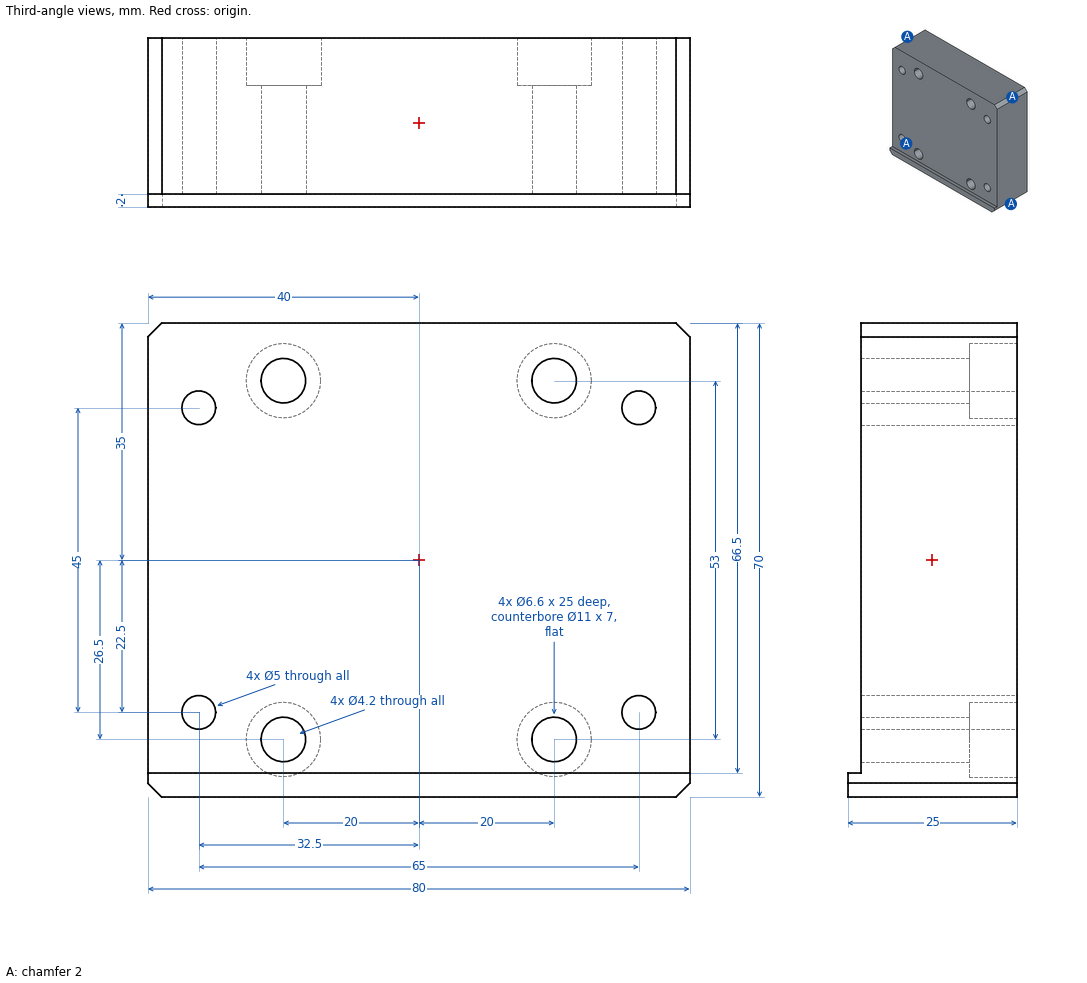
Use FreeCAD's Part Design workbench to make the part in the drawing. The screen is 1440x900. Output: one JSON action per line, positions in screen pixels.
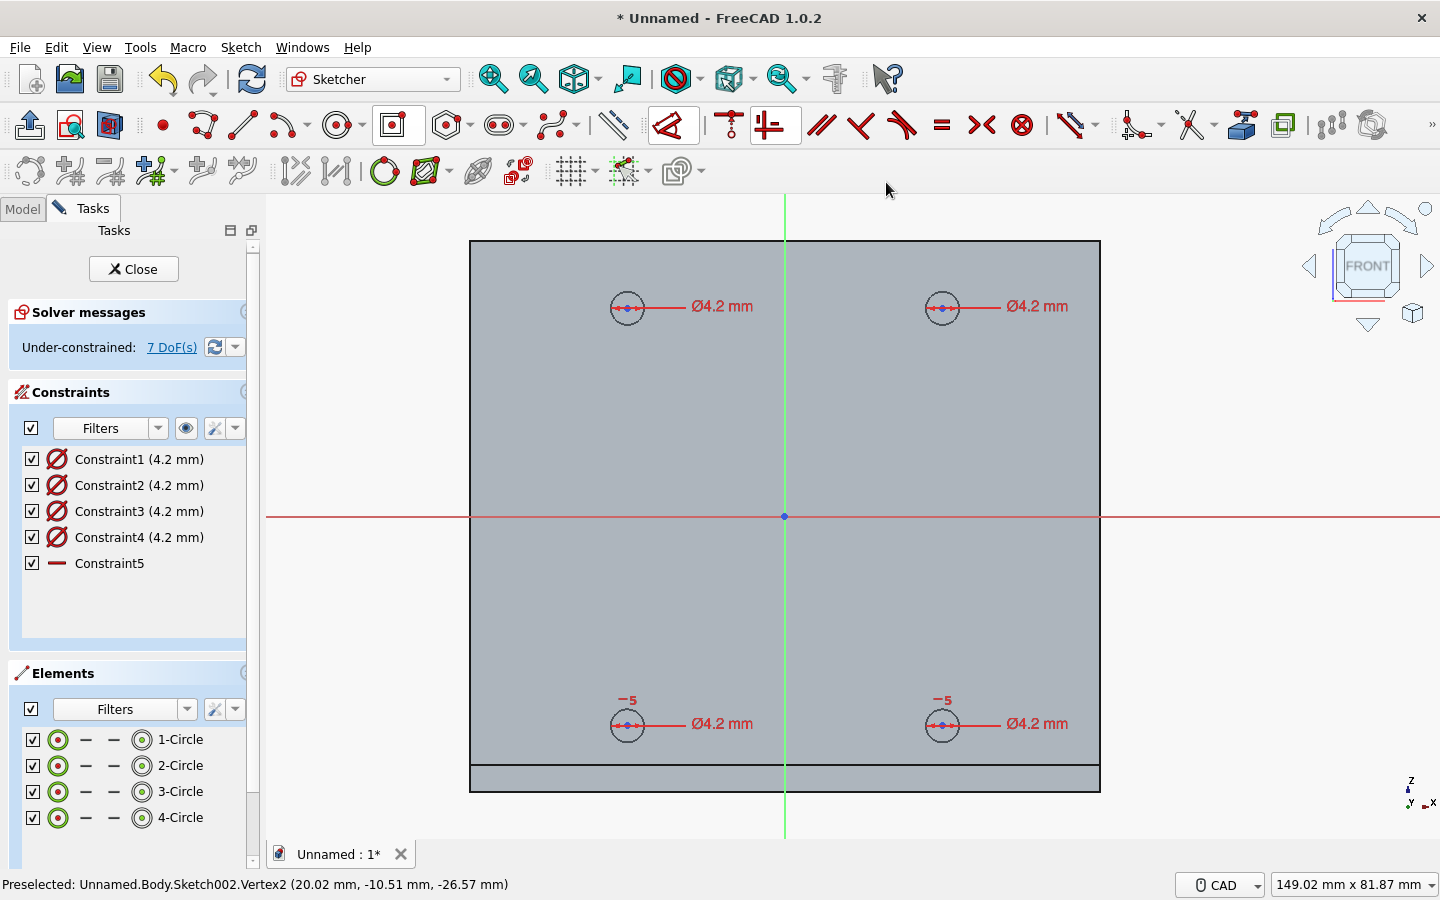
{"action": "left_click", "coordinate": [943, 726]}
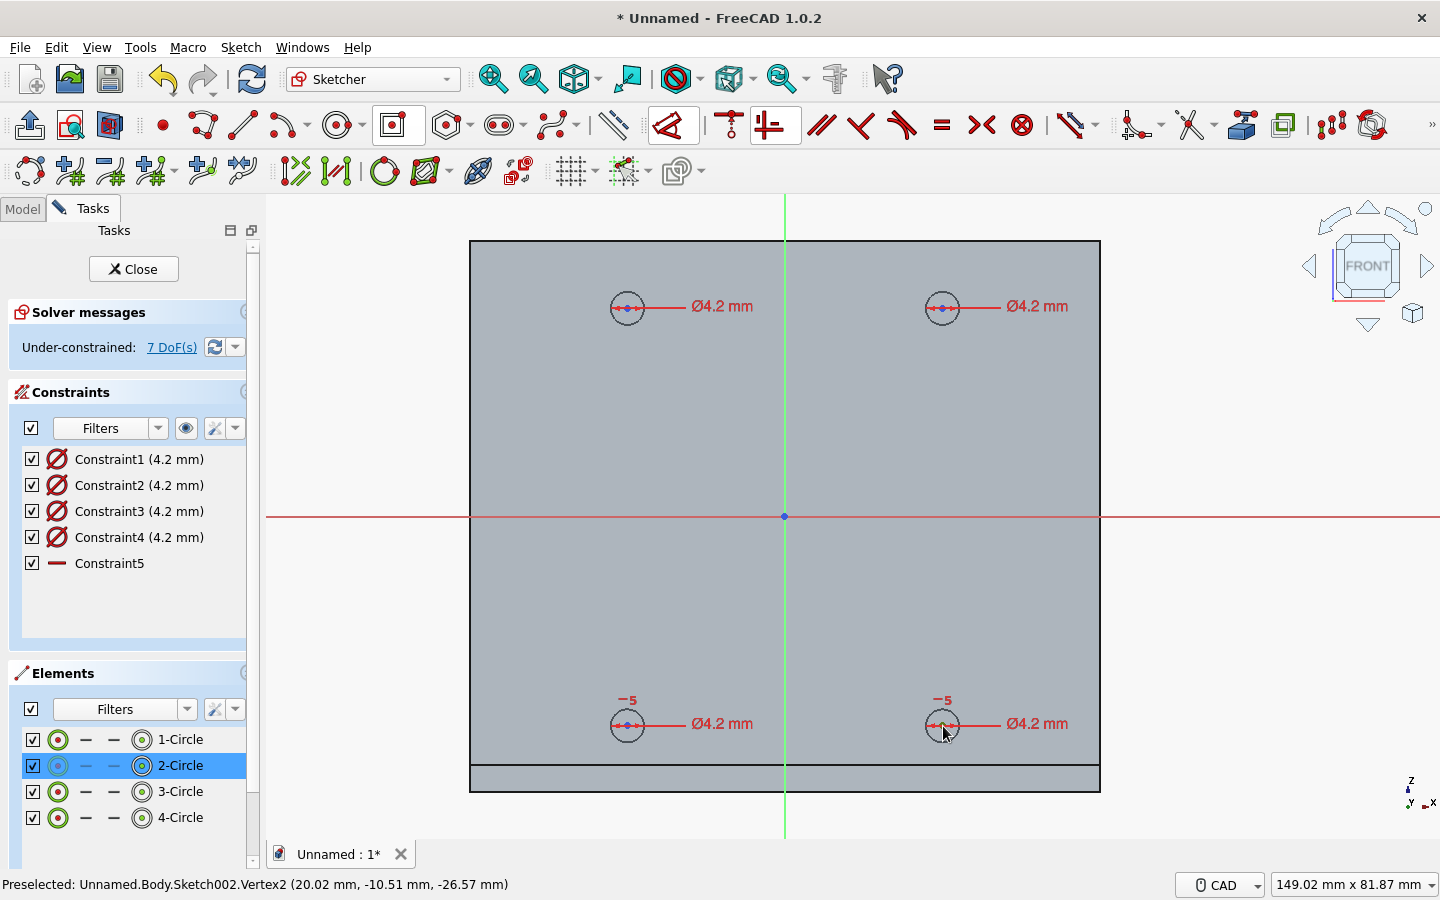
{"action": "left_click", "coordinate": [943, 308]}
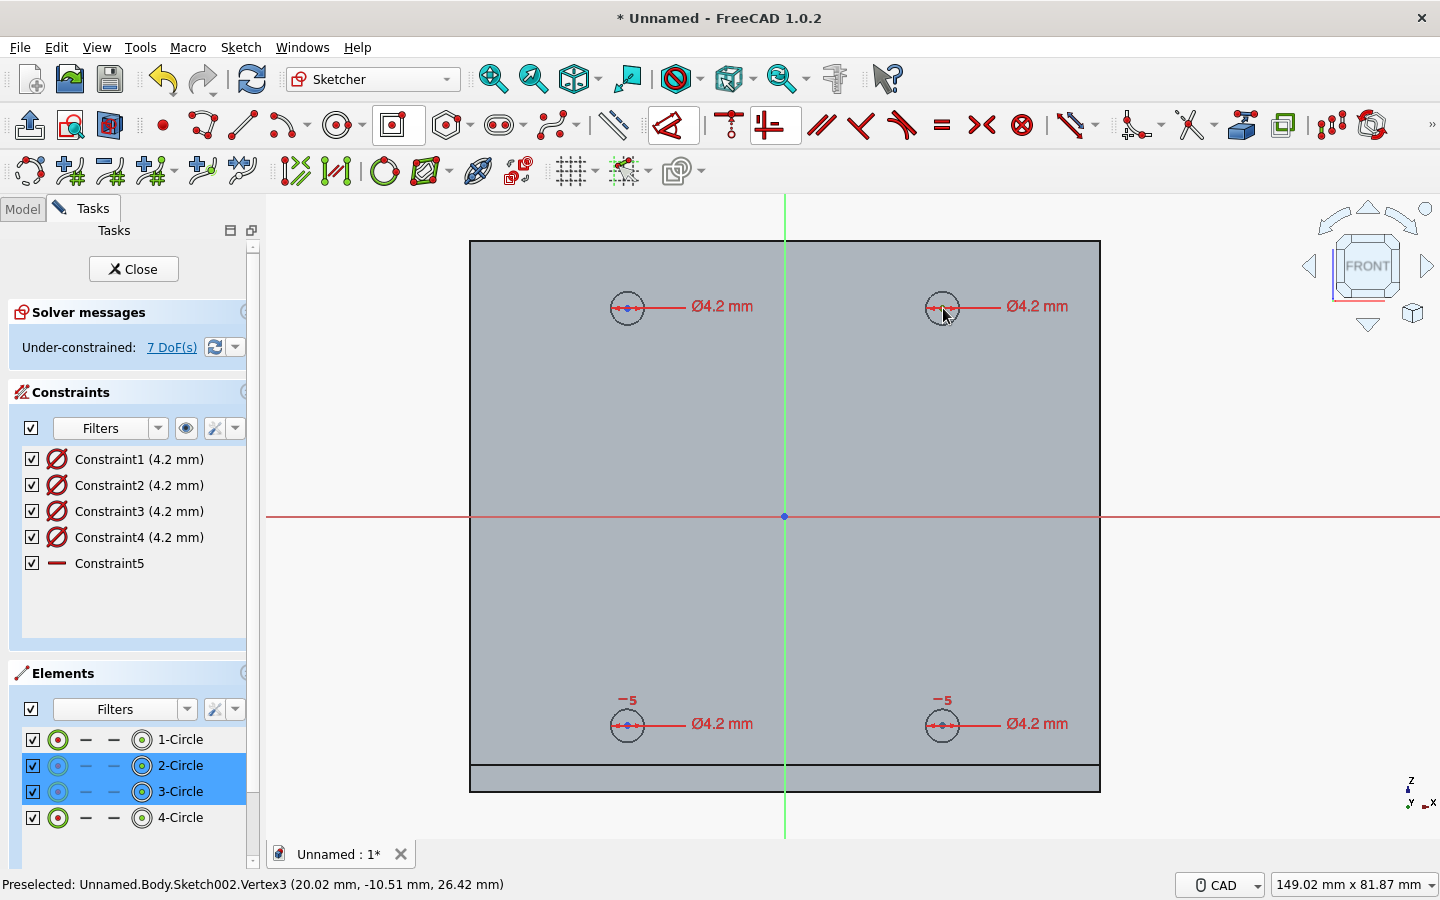
{"action": "left_click", "coordinate": [796, 126]}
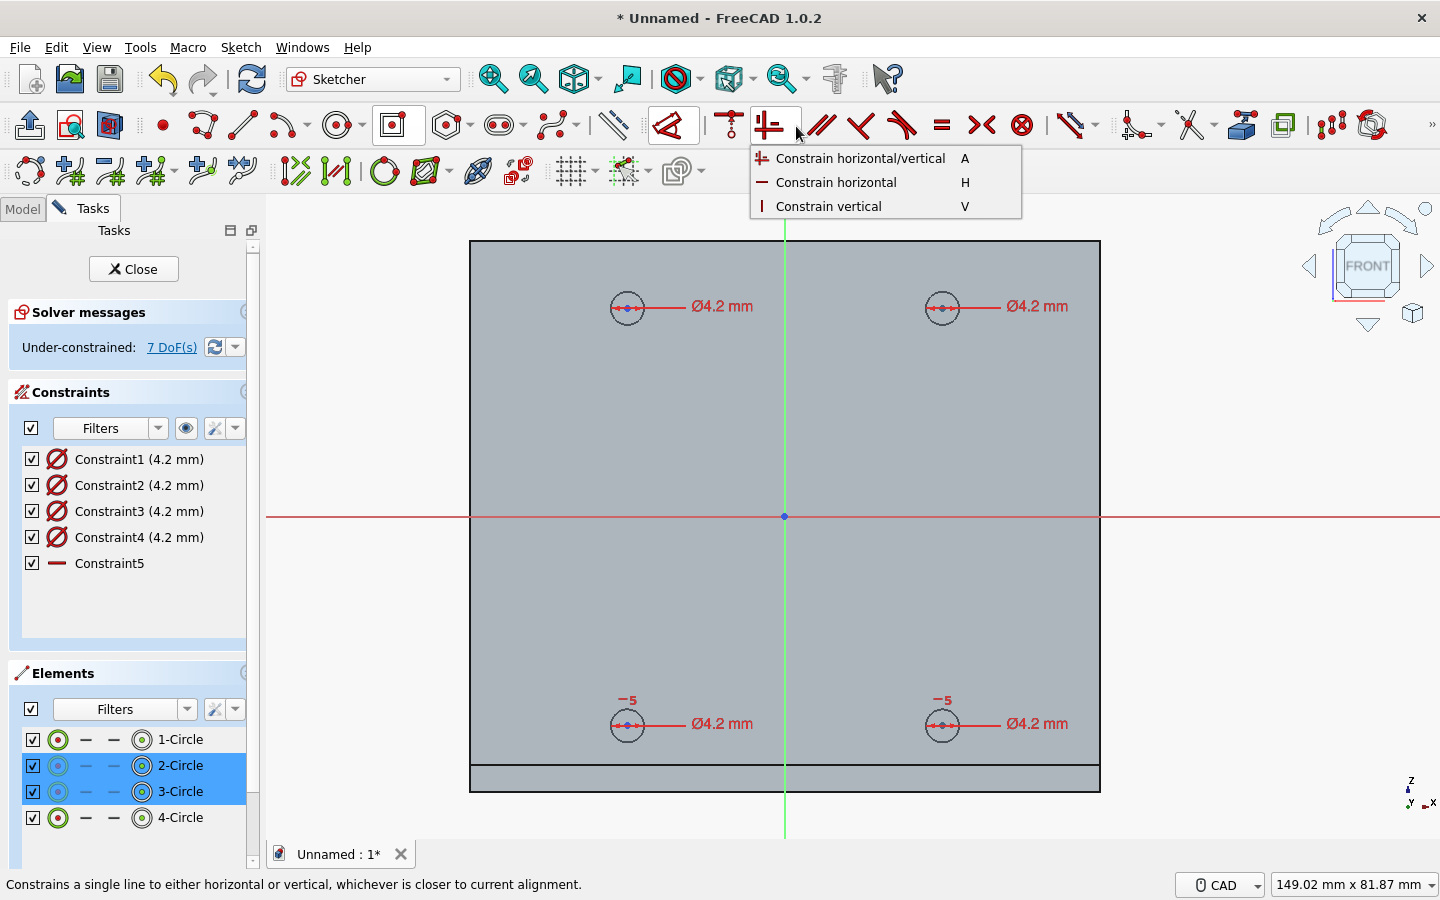
{"action": "left_click", "coordinate": [886, 206]}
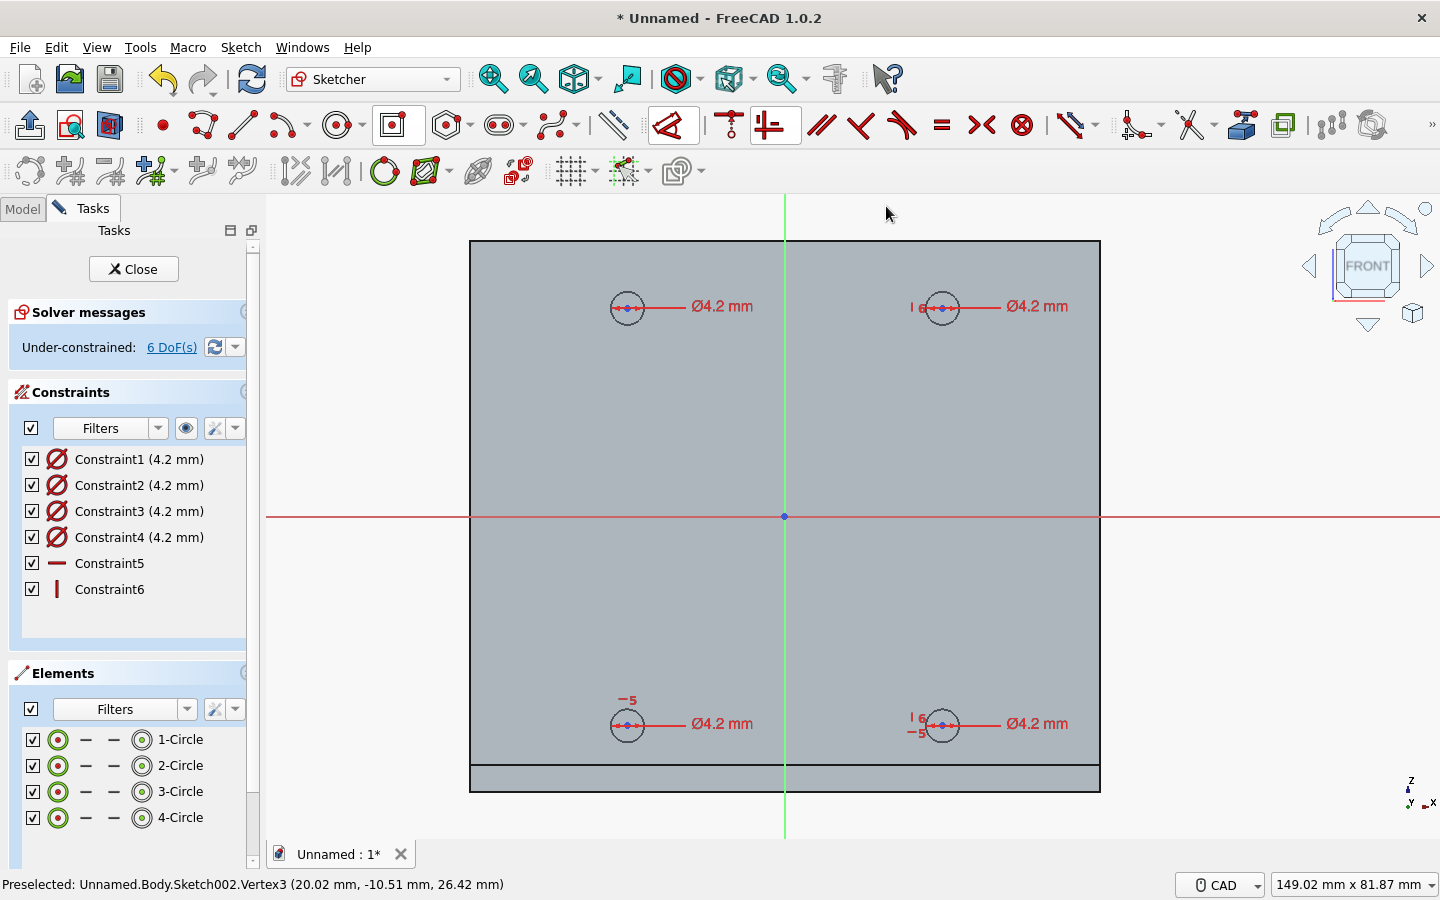
{"action": "left_click", "coordinate": [627, 726]}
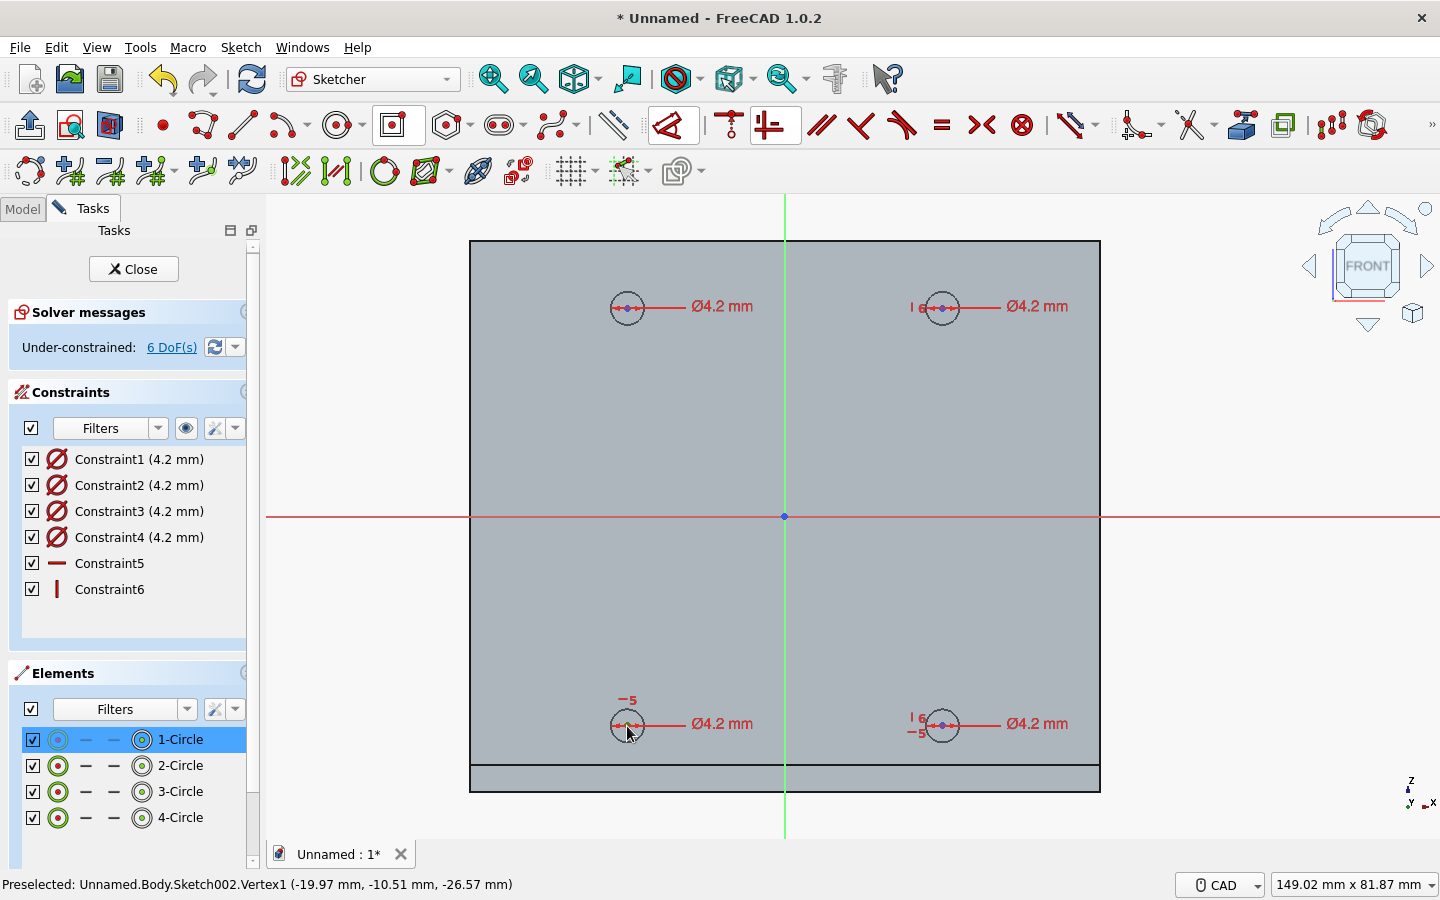
{"action": "left_click", "coordinate": [627, 308]}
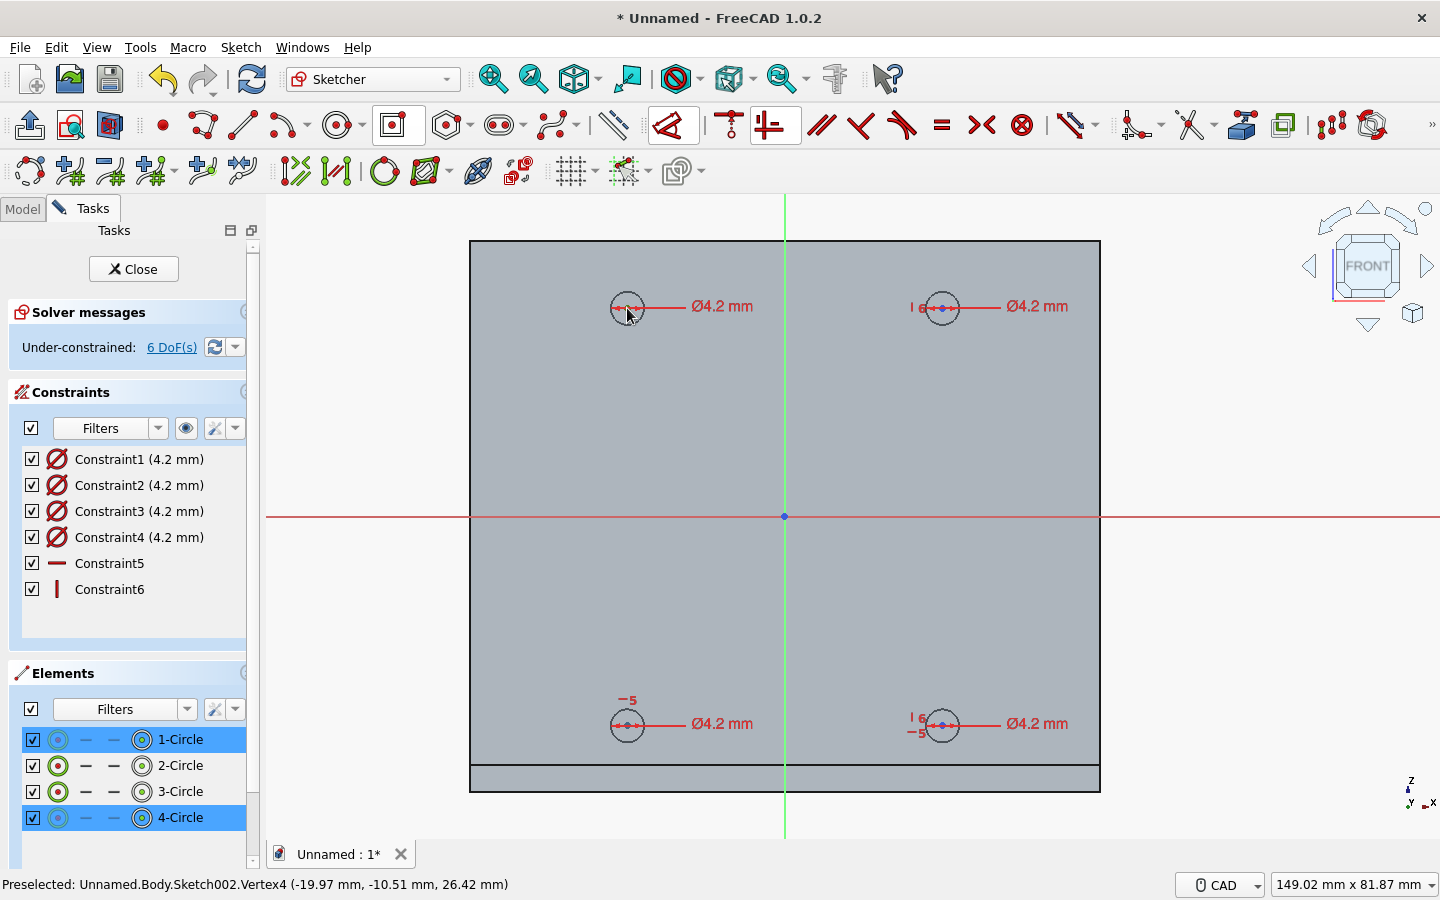
{"action": "key", "text": "v"}